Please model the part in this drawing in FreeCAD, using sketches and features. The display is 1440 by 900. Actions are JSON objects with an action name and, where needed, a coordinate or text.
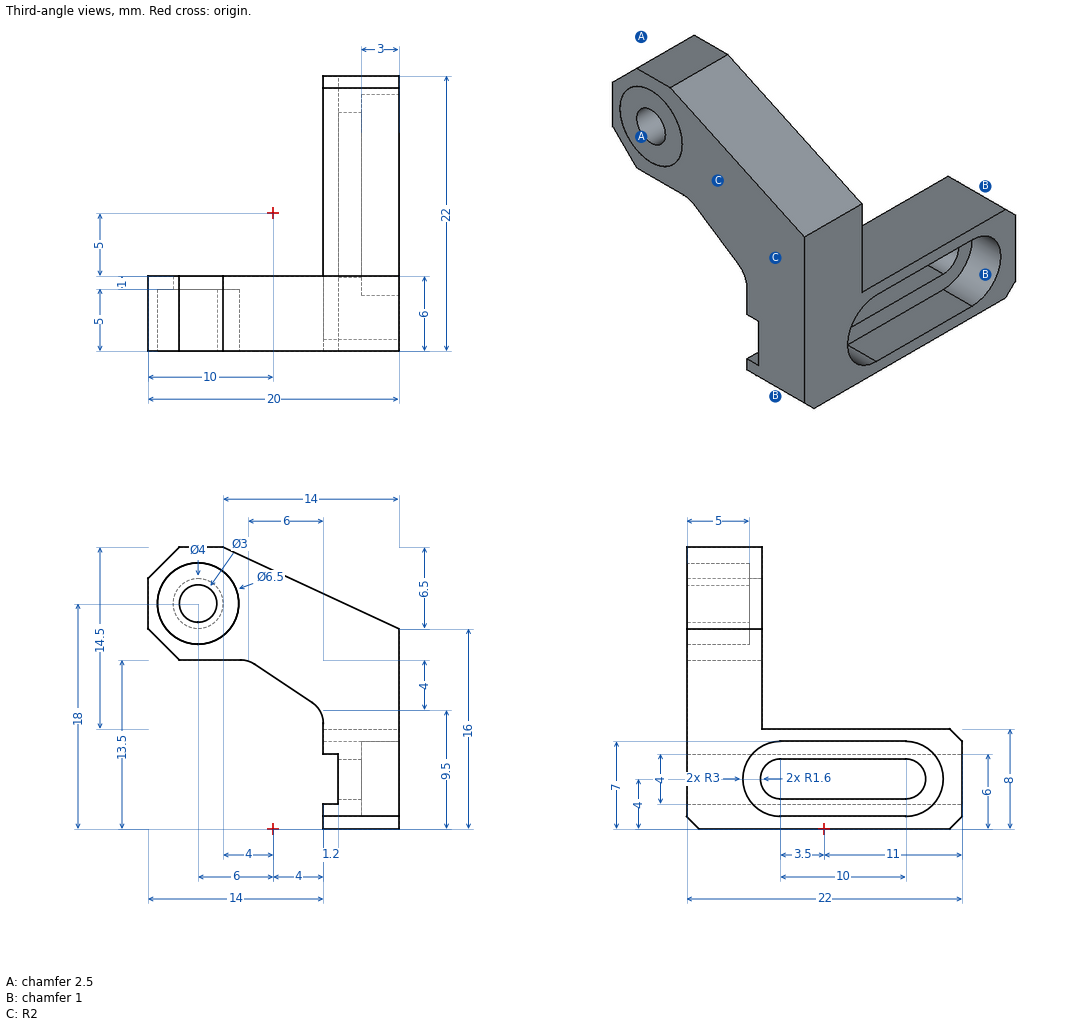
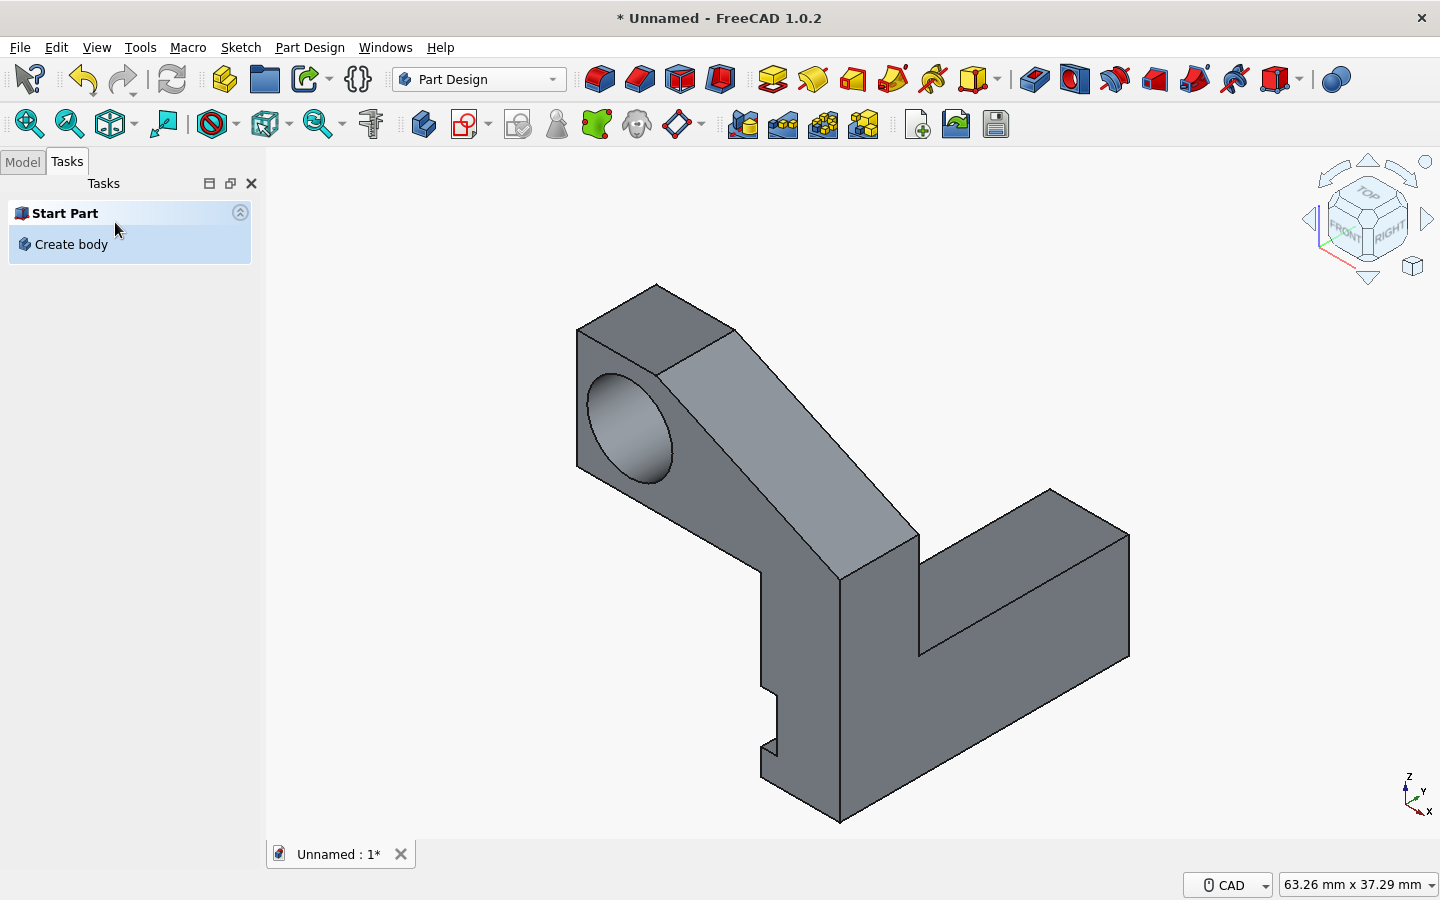
{"action": "left_click", "coordinate": [1067, 639]}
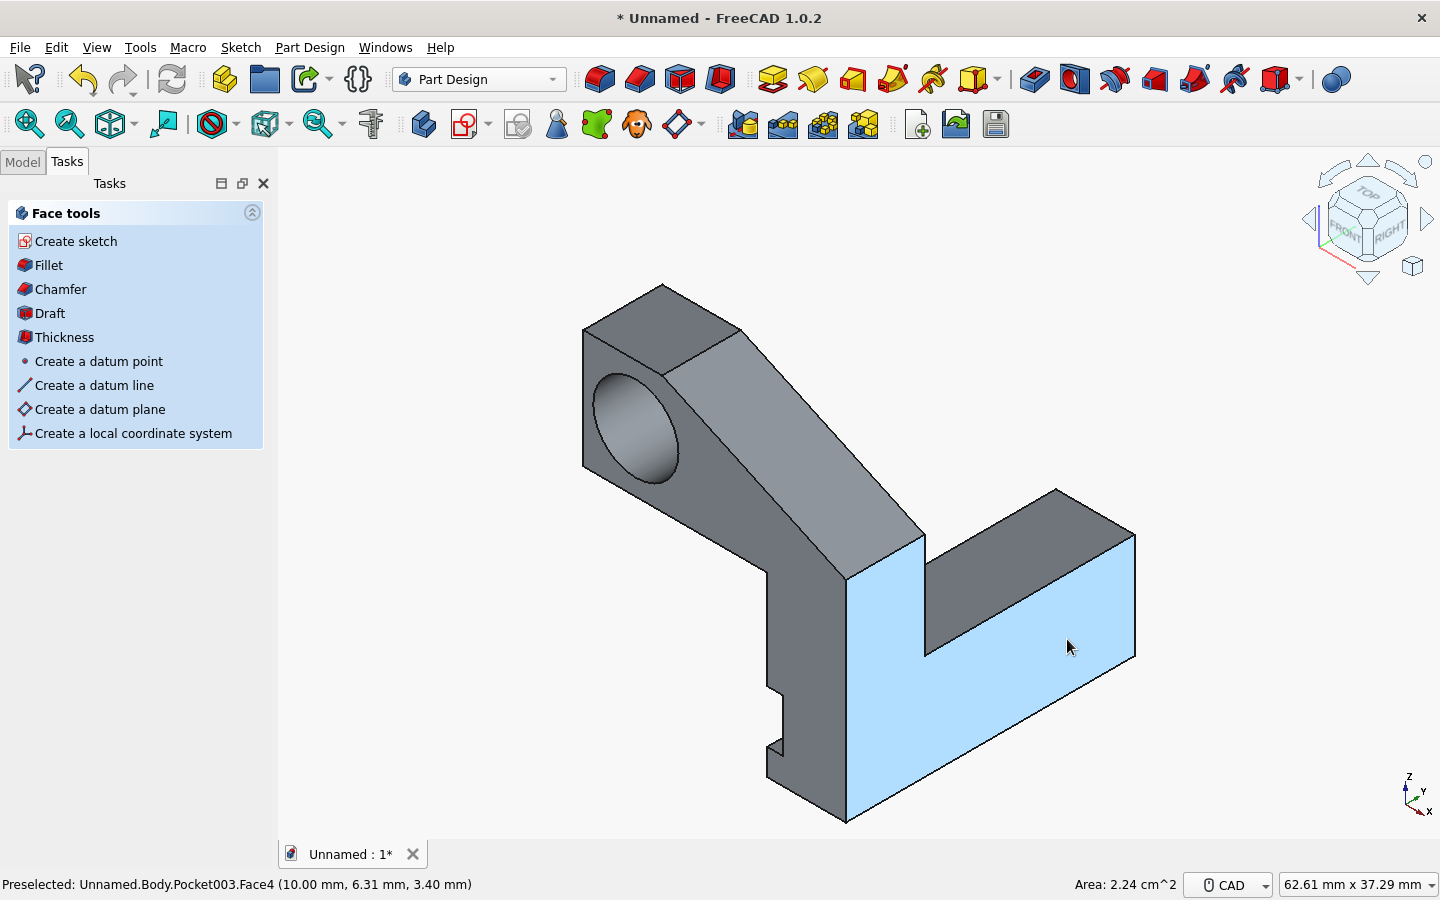
{"action": "left_click", "coordinate": [464, 124]}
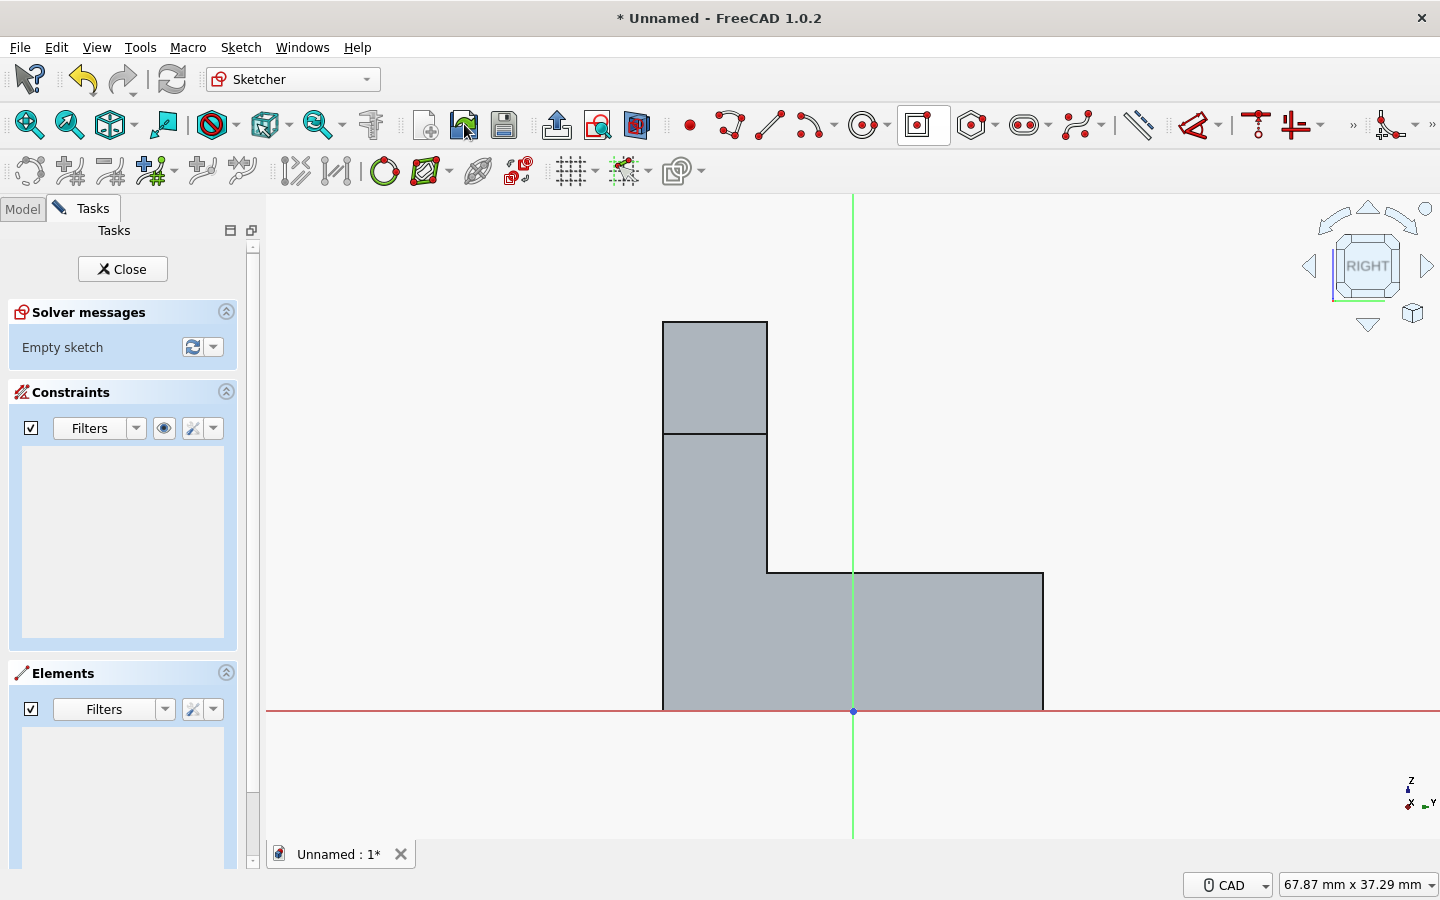
{"action": "scroll", "coordinate": [920, 726], "scroll_direction": "up", "scroll_amount": 6}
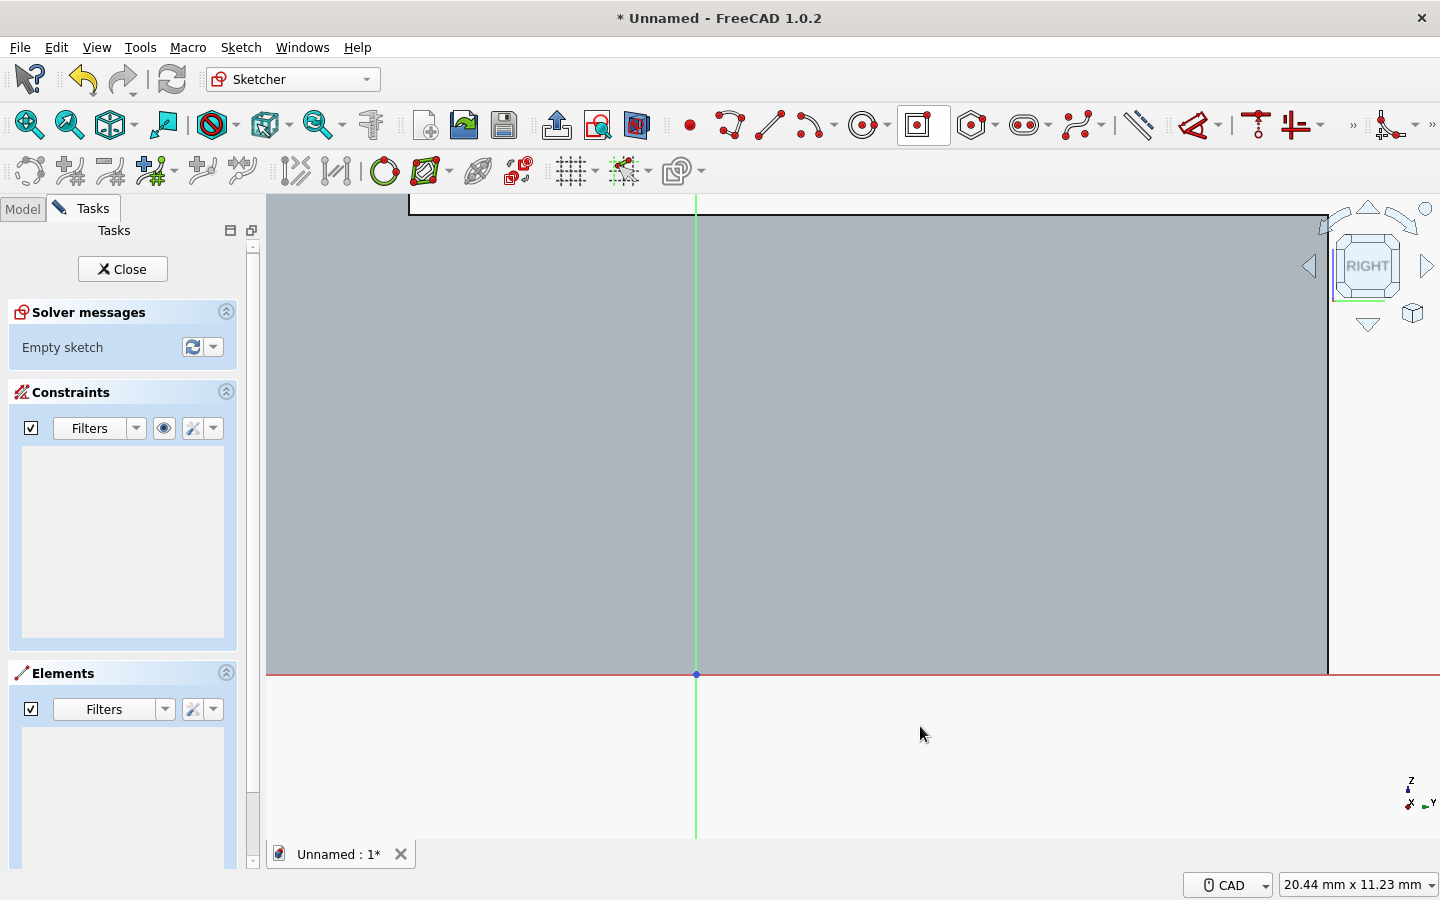
{"action": "left_click", "coordinate": [1024, 126]}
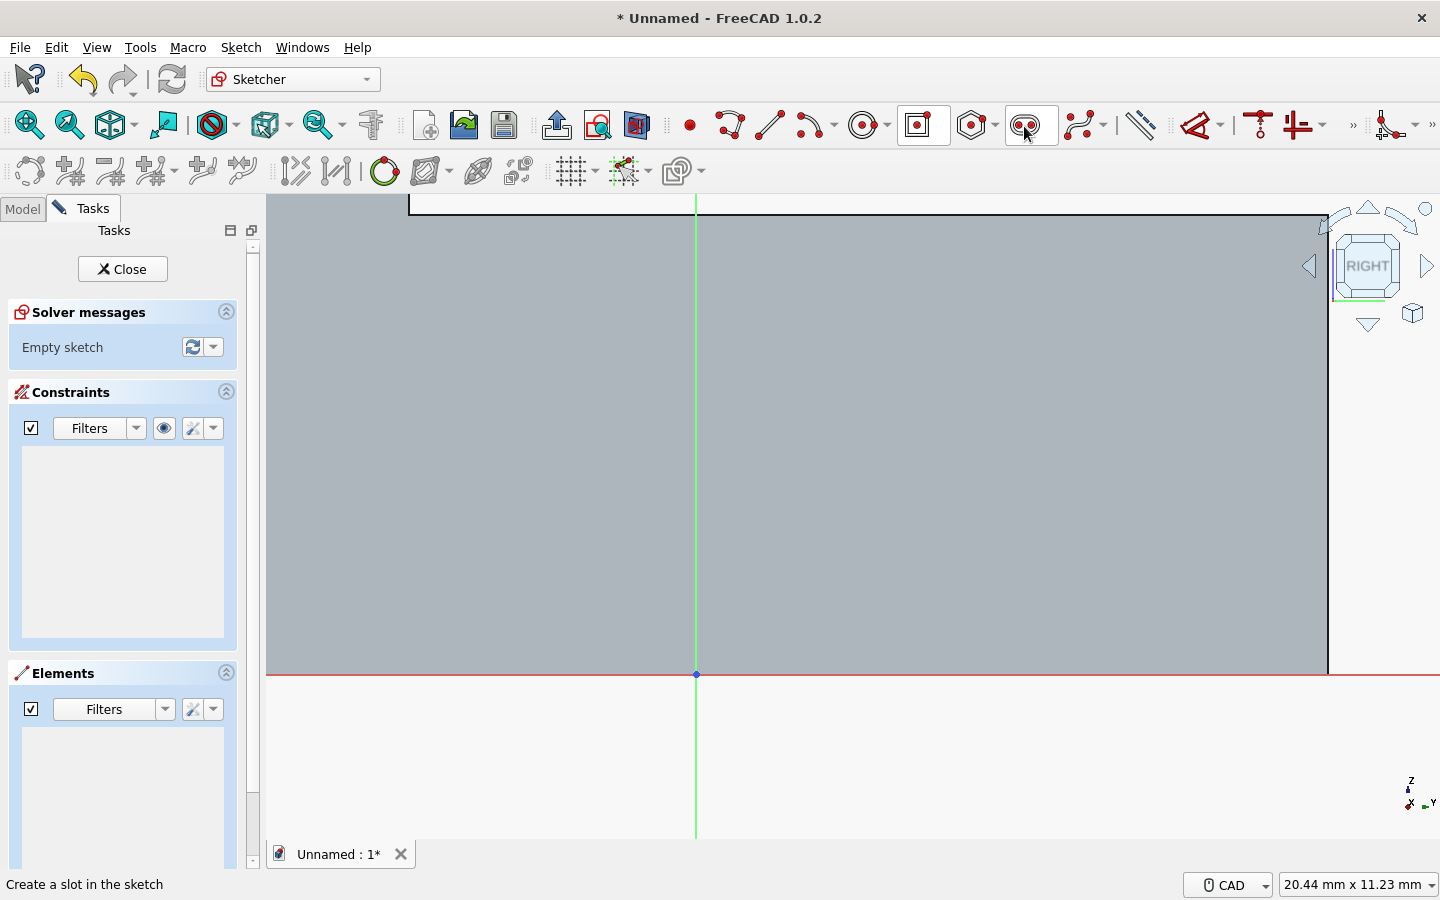
{"action": "left_click", "coordinate": [495, 445]}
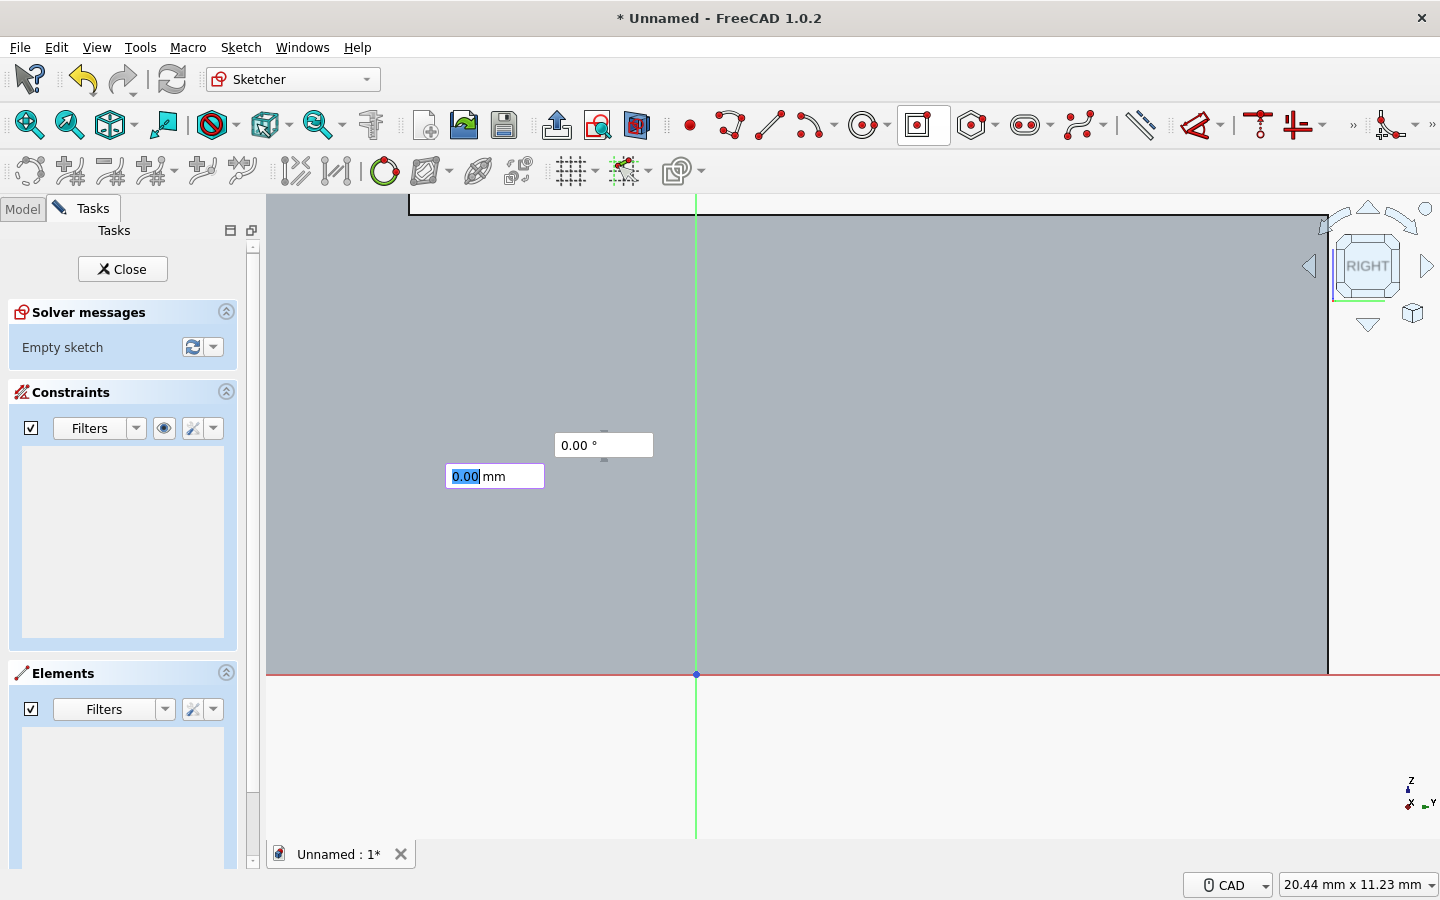
{"action": "left_click", "coordinate": [1070, 445]}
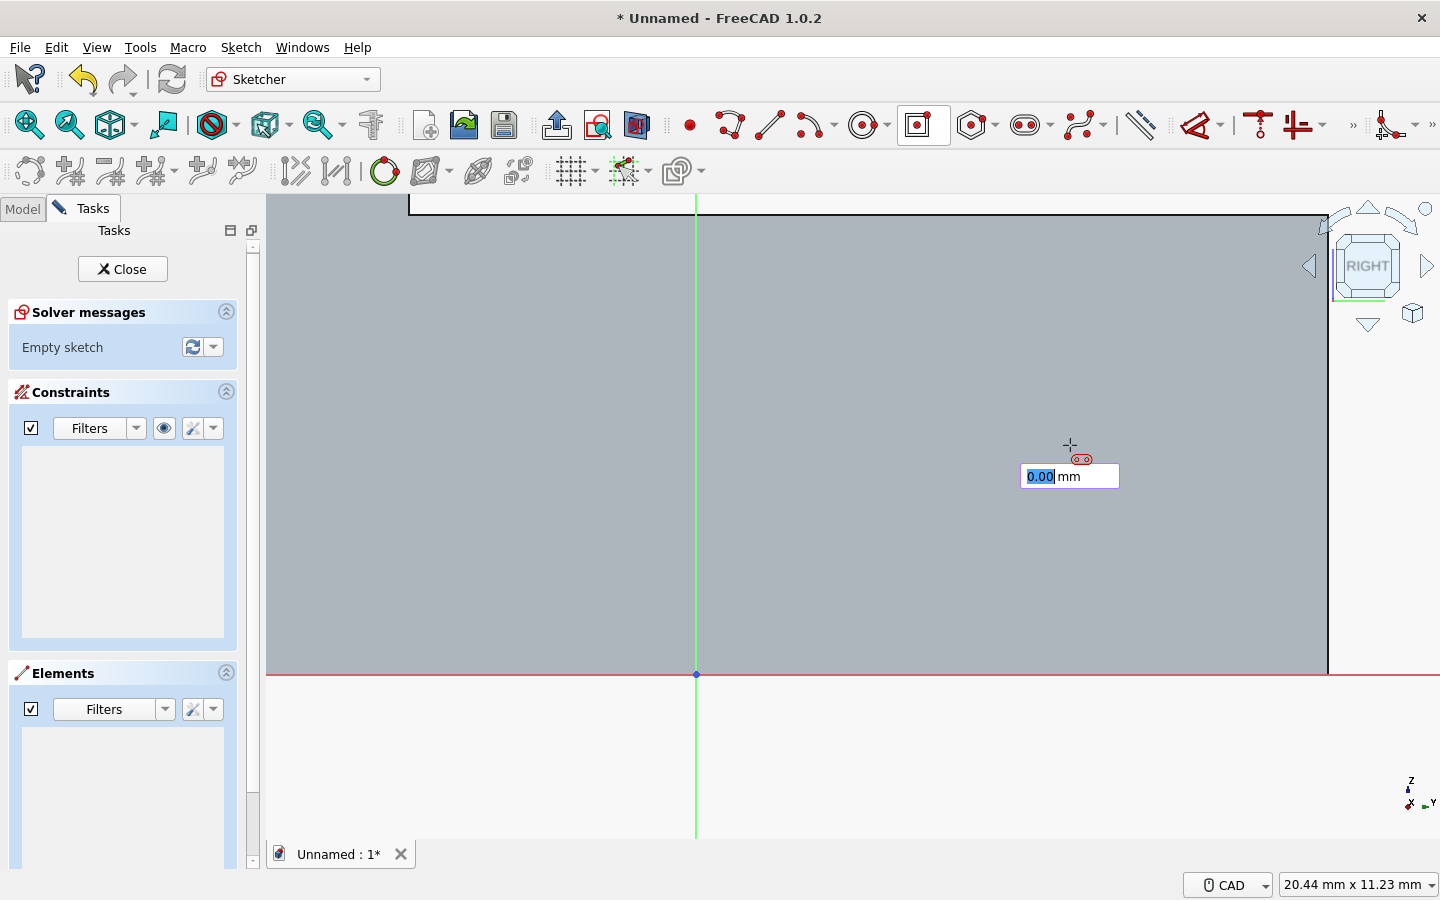
{"action": "left_click", "coordinate": [782, 353]}
{"action": "key", "text": "Escape"}